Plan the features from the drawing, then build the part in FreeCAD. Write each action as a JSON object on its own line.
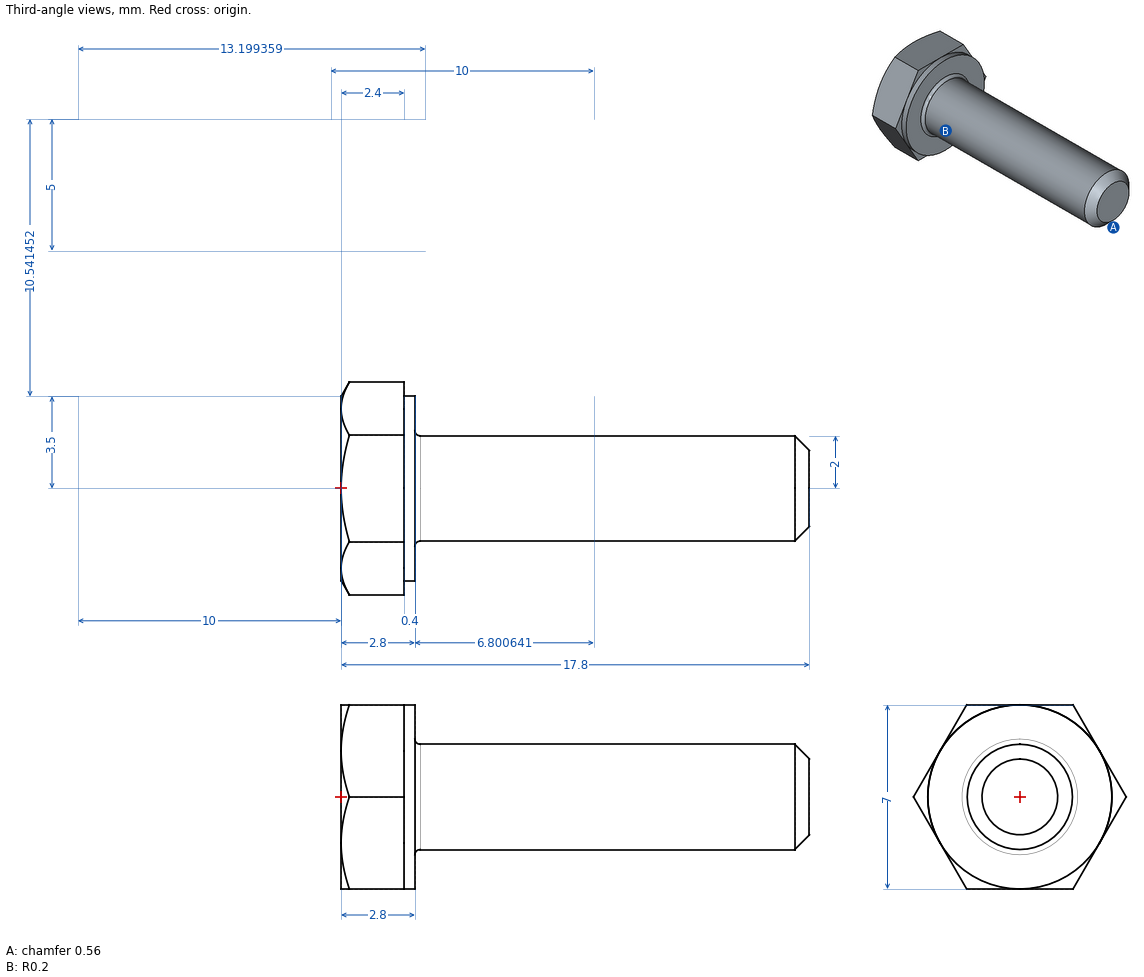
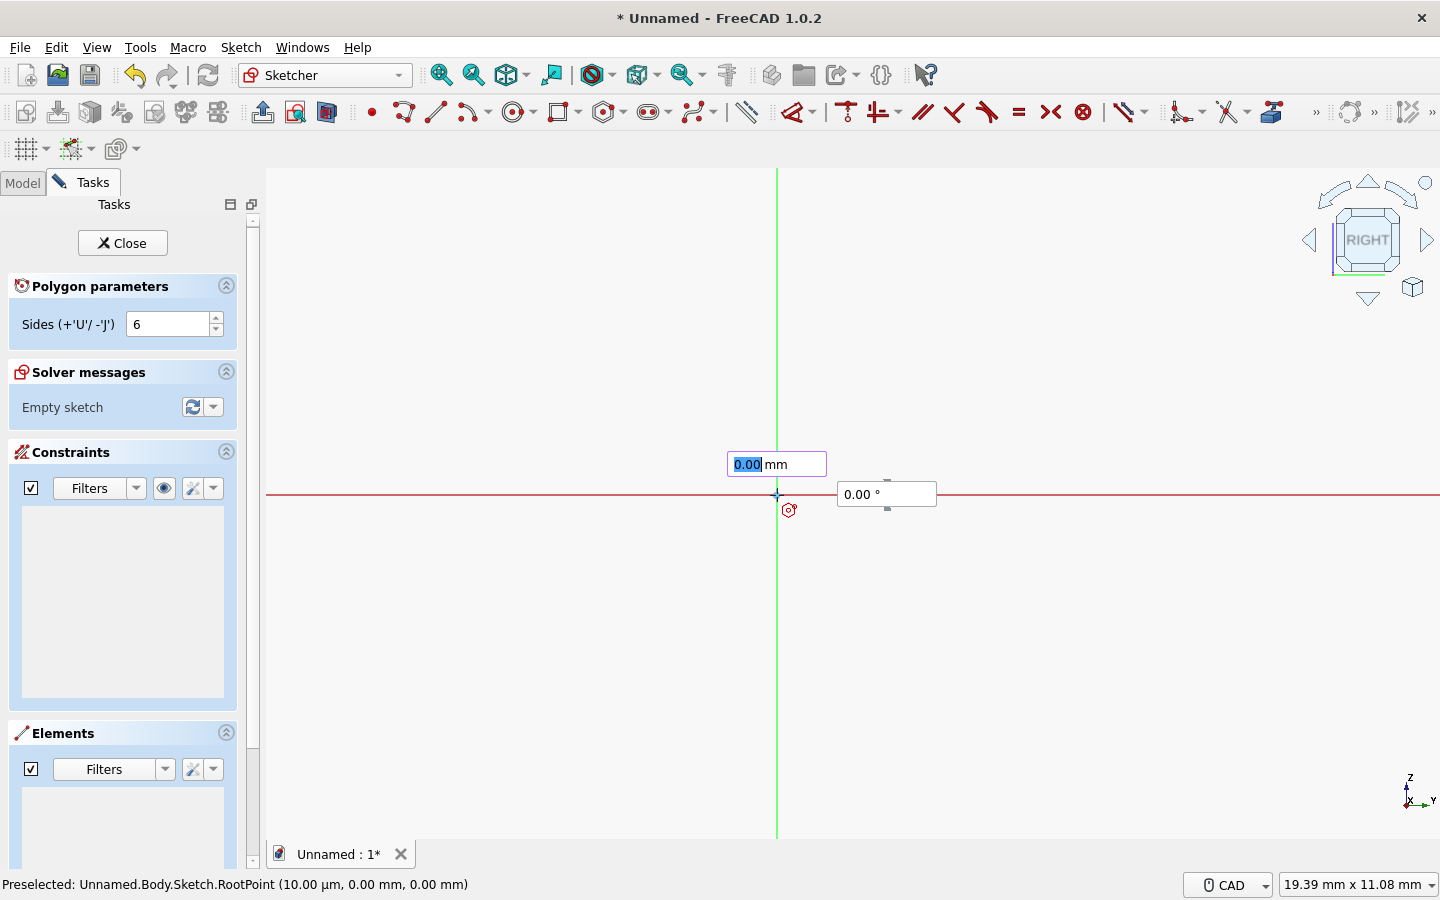
{"action": "left_click", "coordinate": [1021, 495]}
{"action": "key", "text": "Escape"}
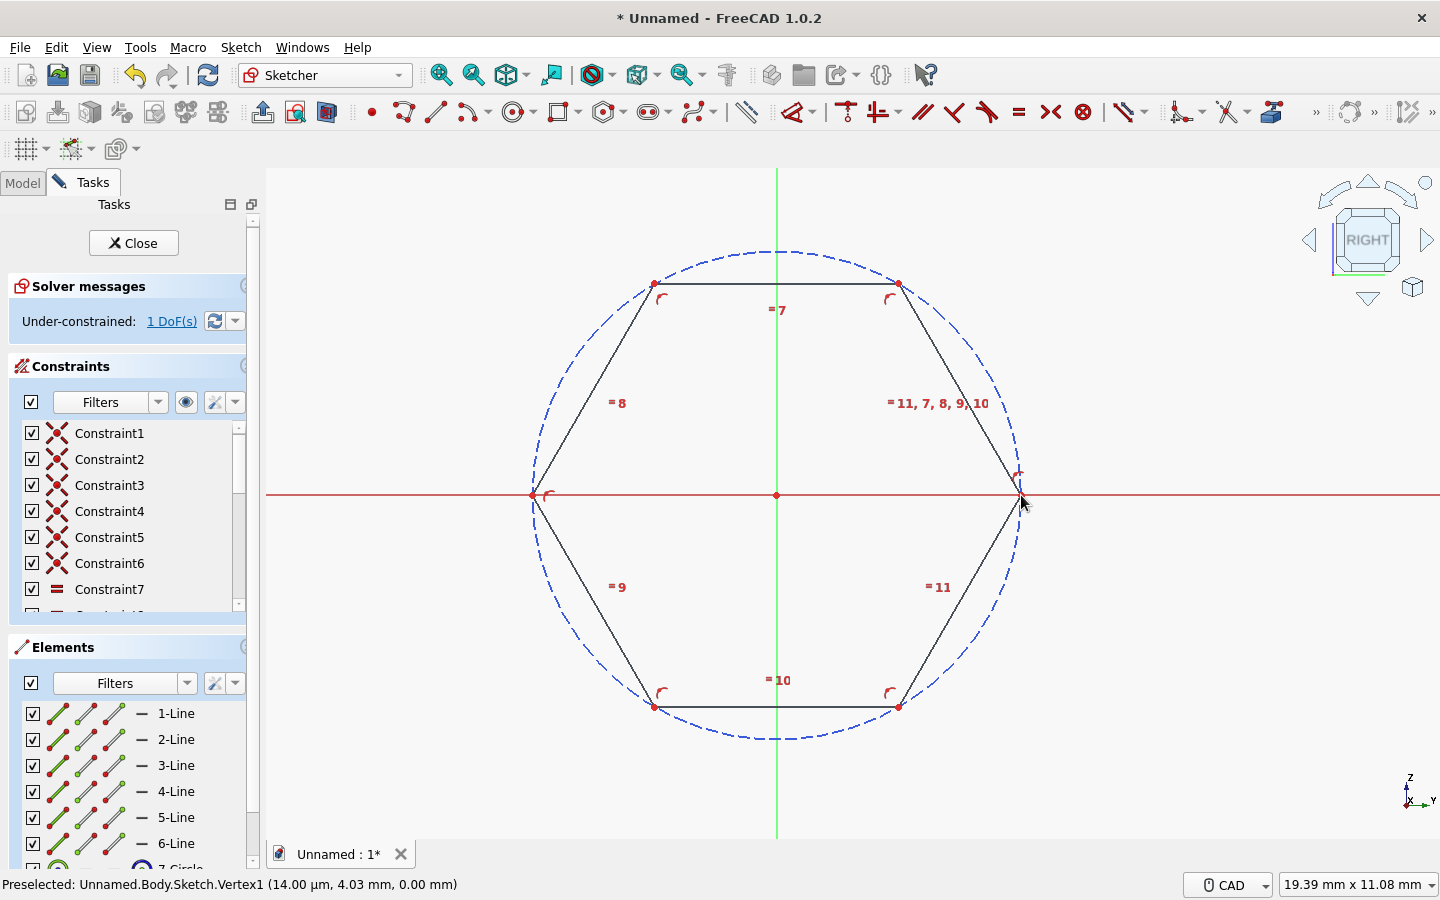
{"action": "key", "text": "d"}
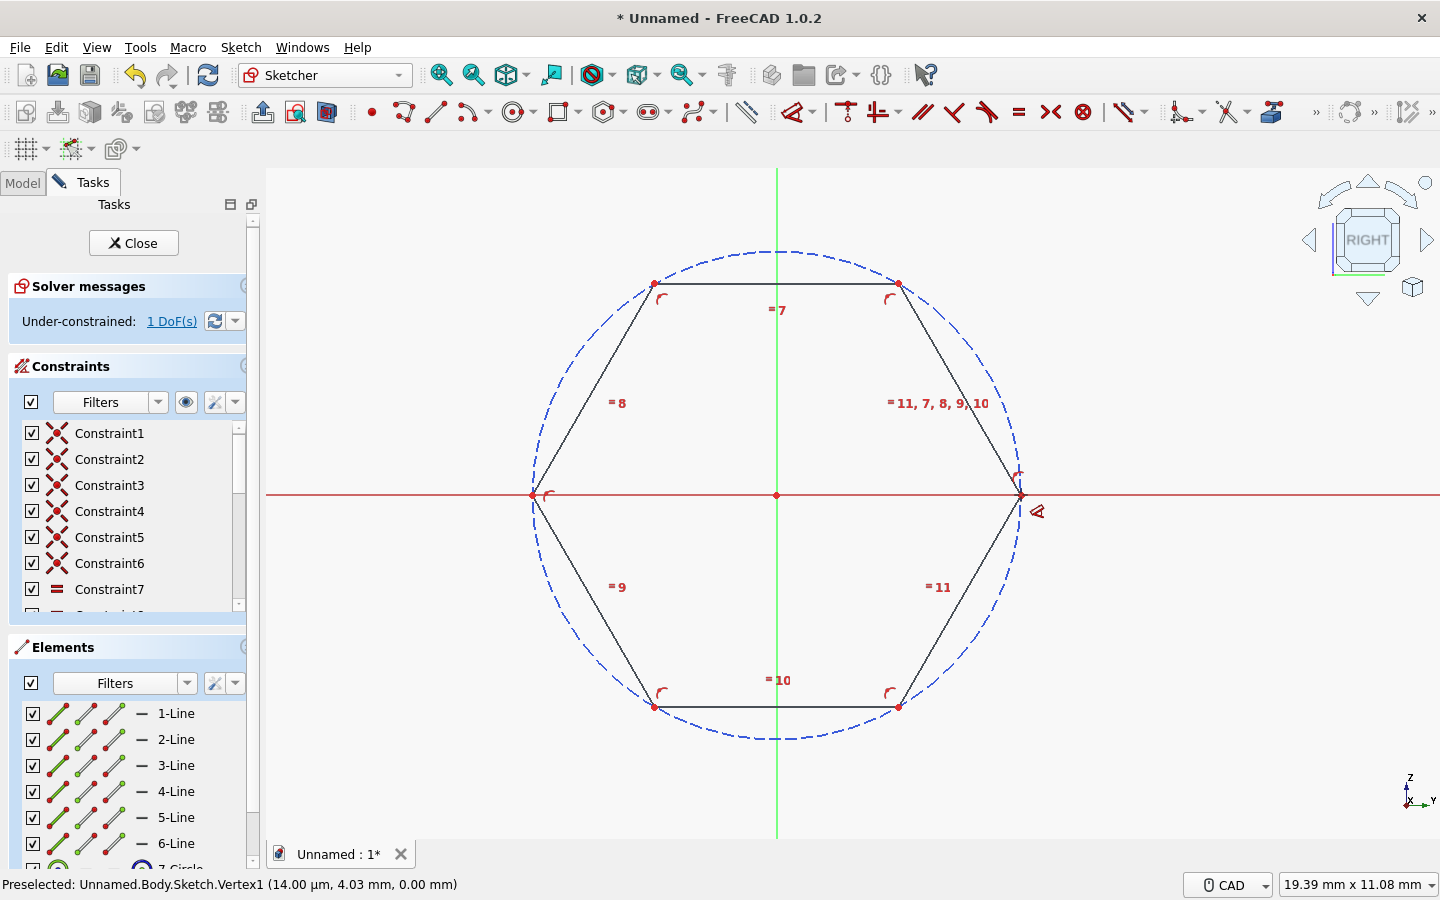
{"action": "left_click", "coordinate": [655, 707]}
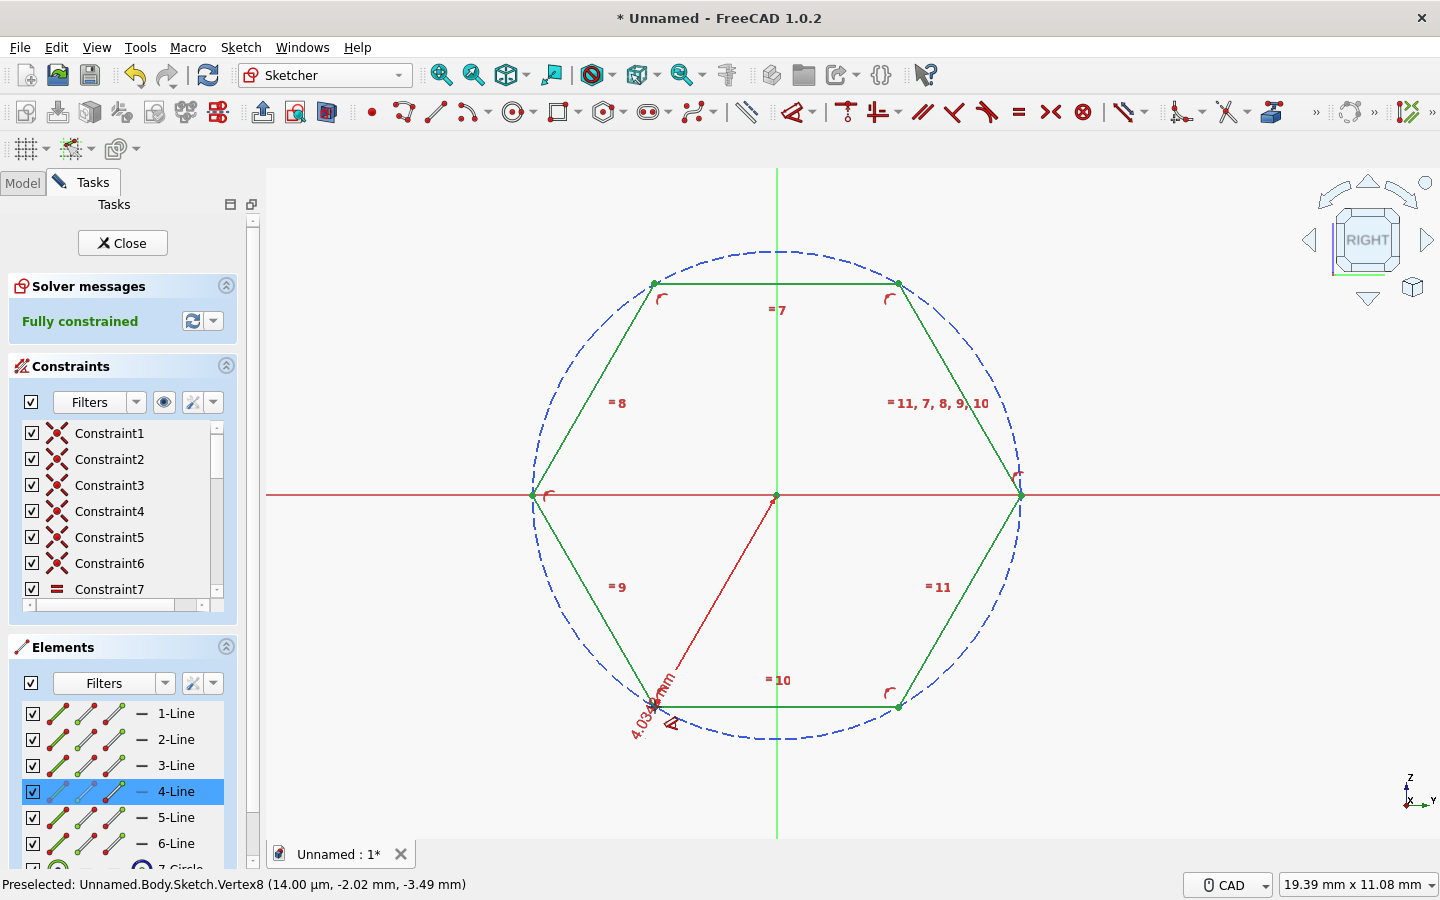
{"action": "left_click", "coordinate": [899, 284]}
{"action": "left_click", "coordinate": [933, 398]}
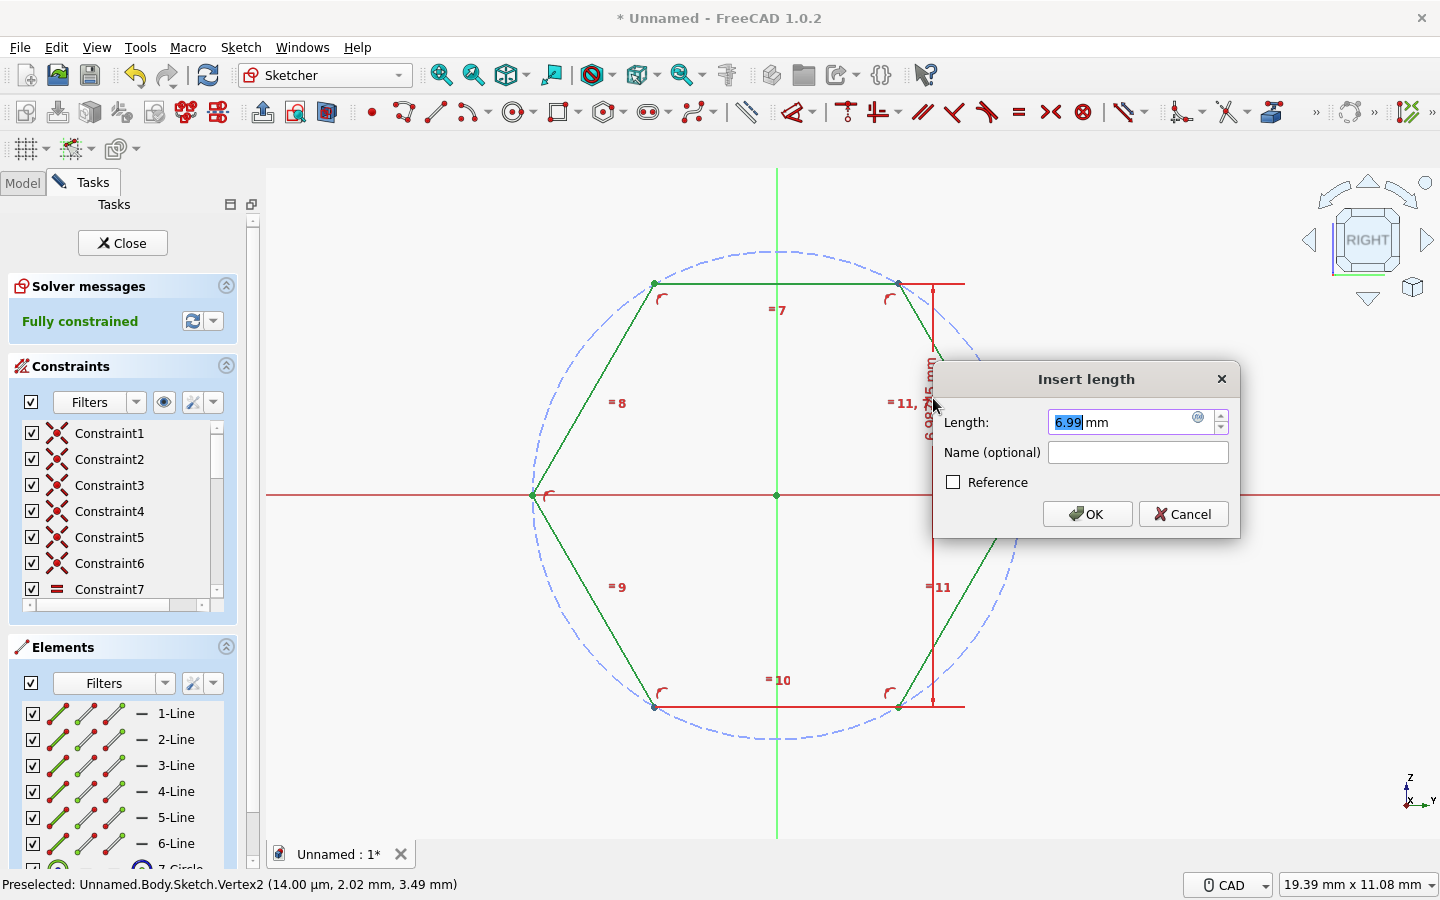
{"action": "type", "text": "7"}
{"action": "key", "text": "Return"}
{"action": "key", "text": "Escape"}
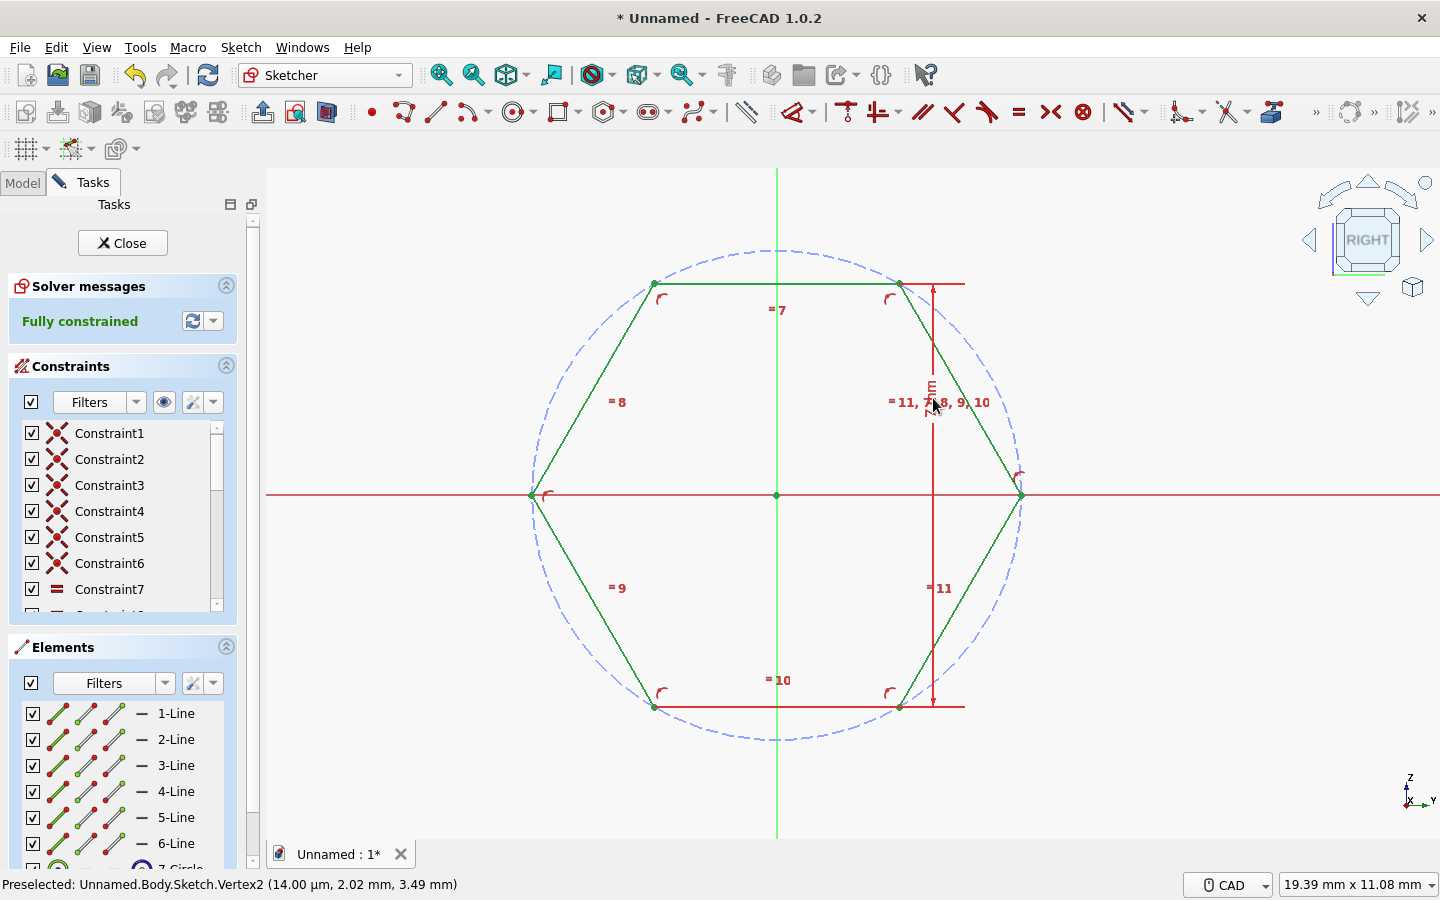
{"action": "left_click", "coordinate": [123, 243]}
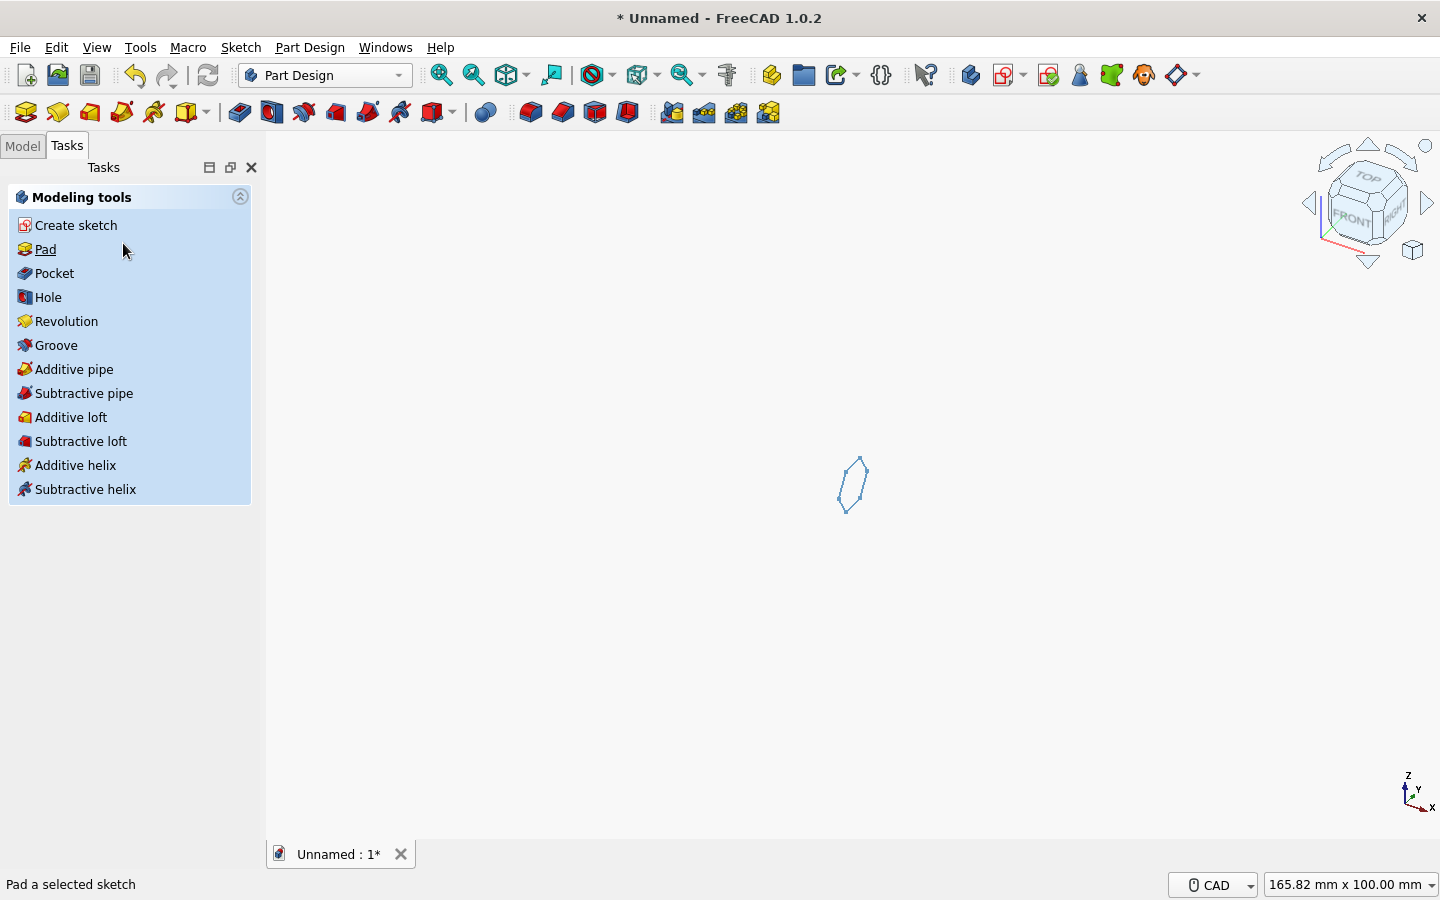
{"action": "left_click", "coordinate": [26, 112]}